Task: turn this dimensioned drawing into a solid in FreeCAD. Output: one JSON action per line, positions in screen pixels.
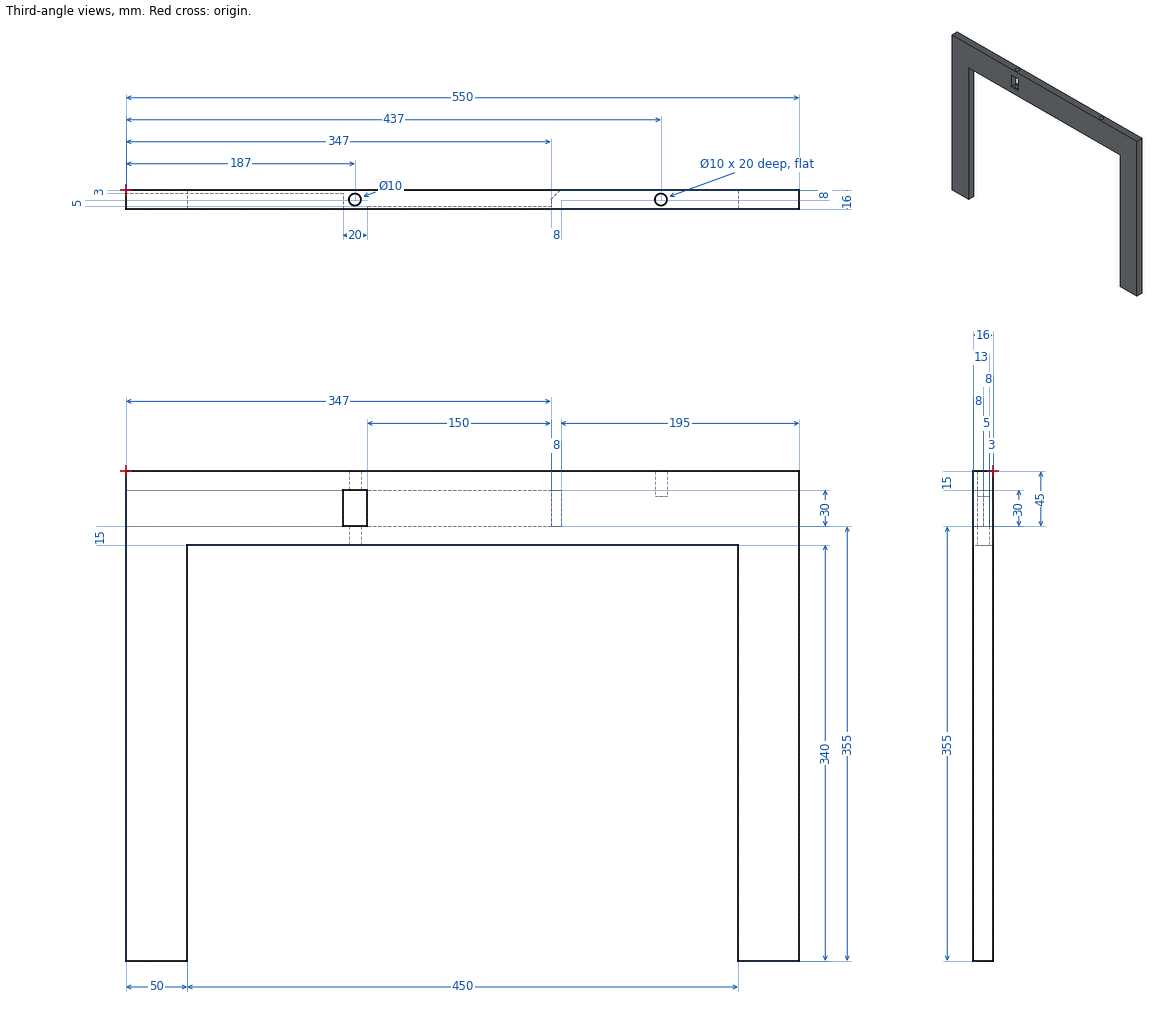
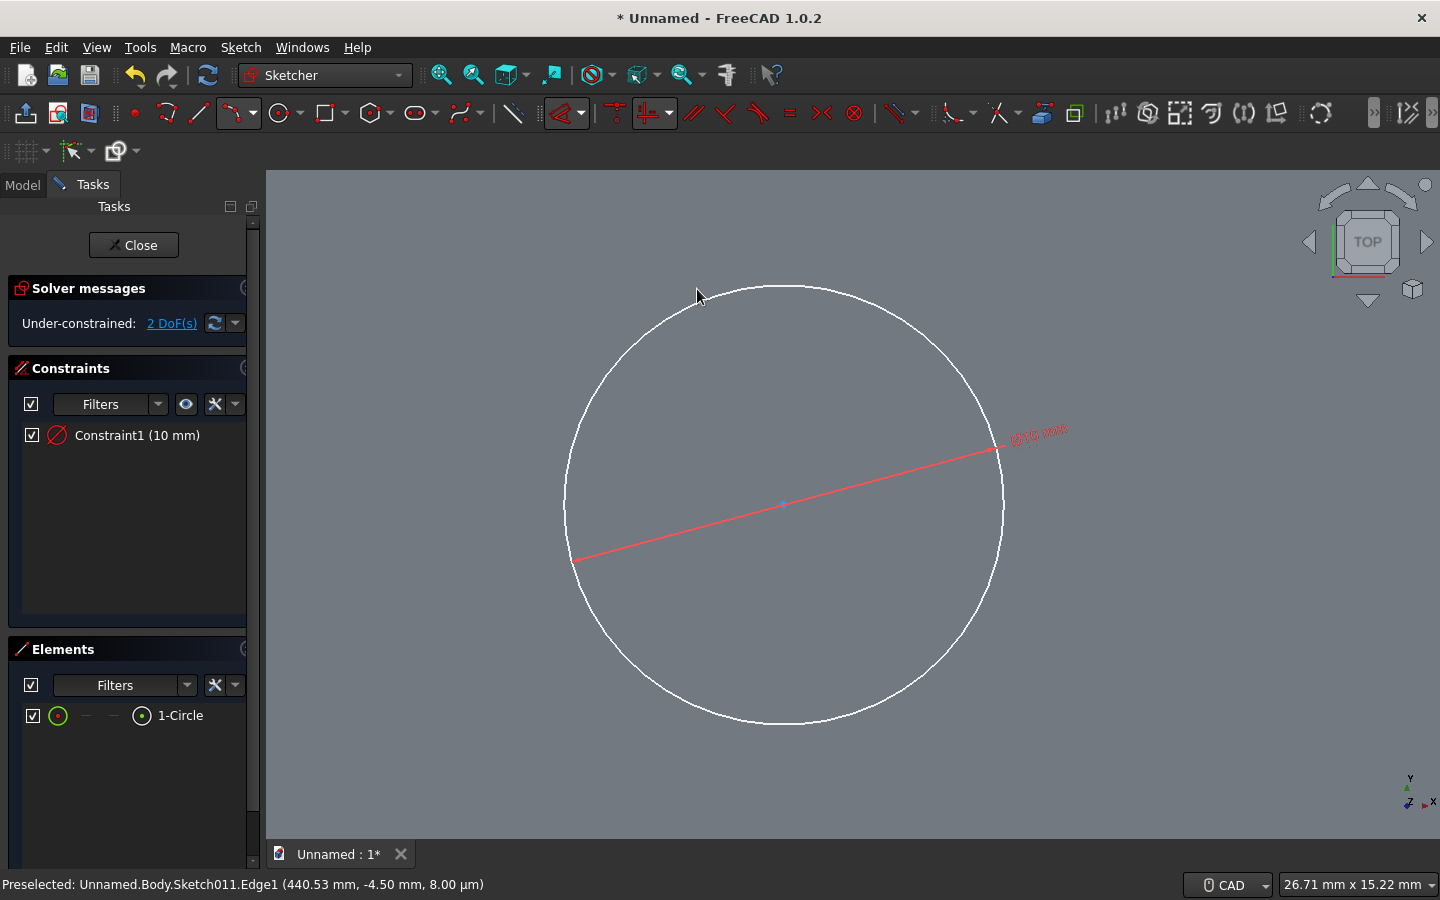
{"action": "left_click", "coordinate": [784, 505]}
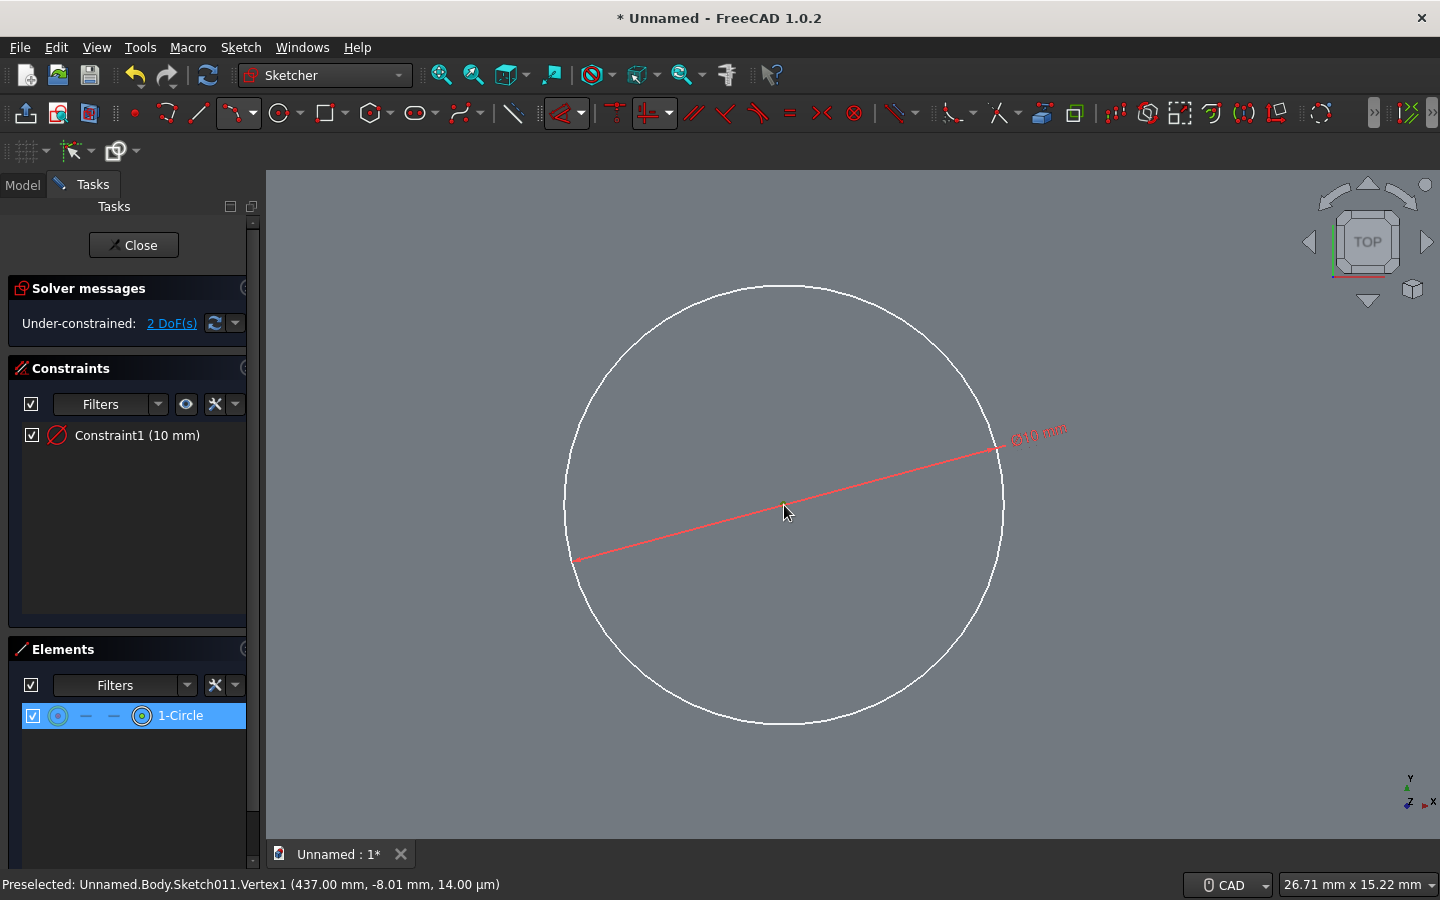
{"action": "left_click", "coordinate": [584, 114]}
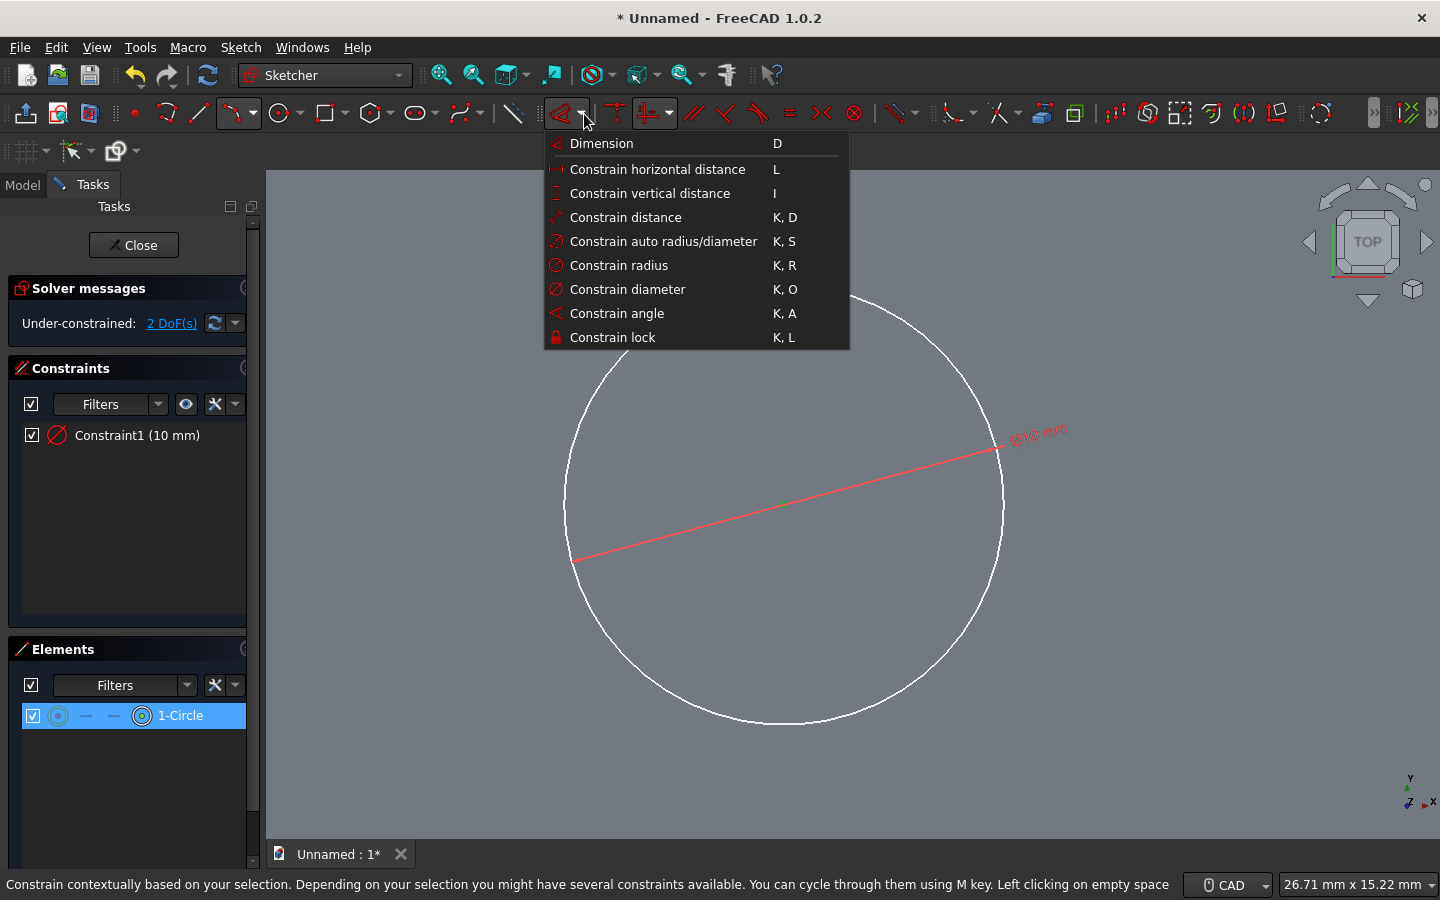
{"action": "left_click", "coordinate": [697, 193]}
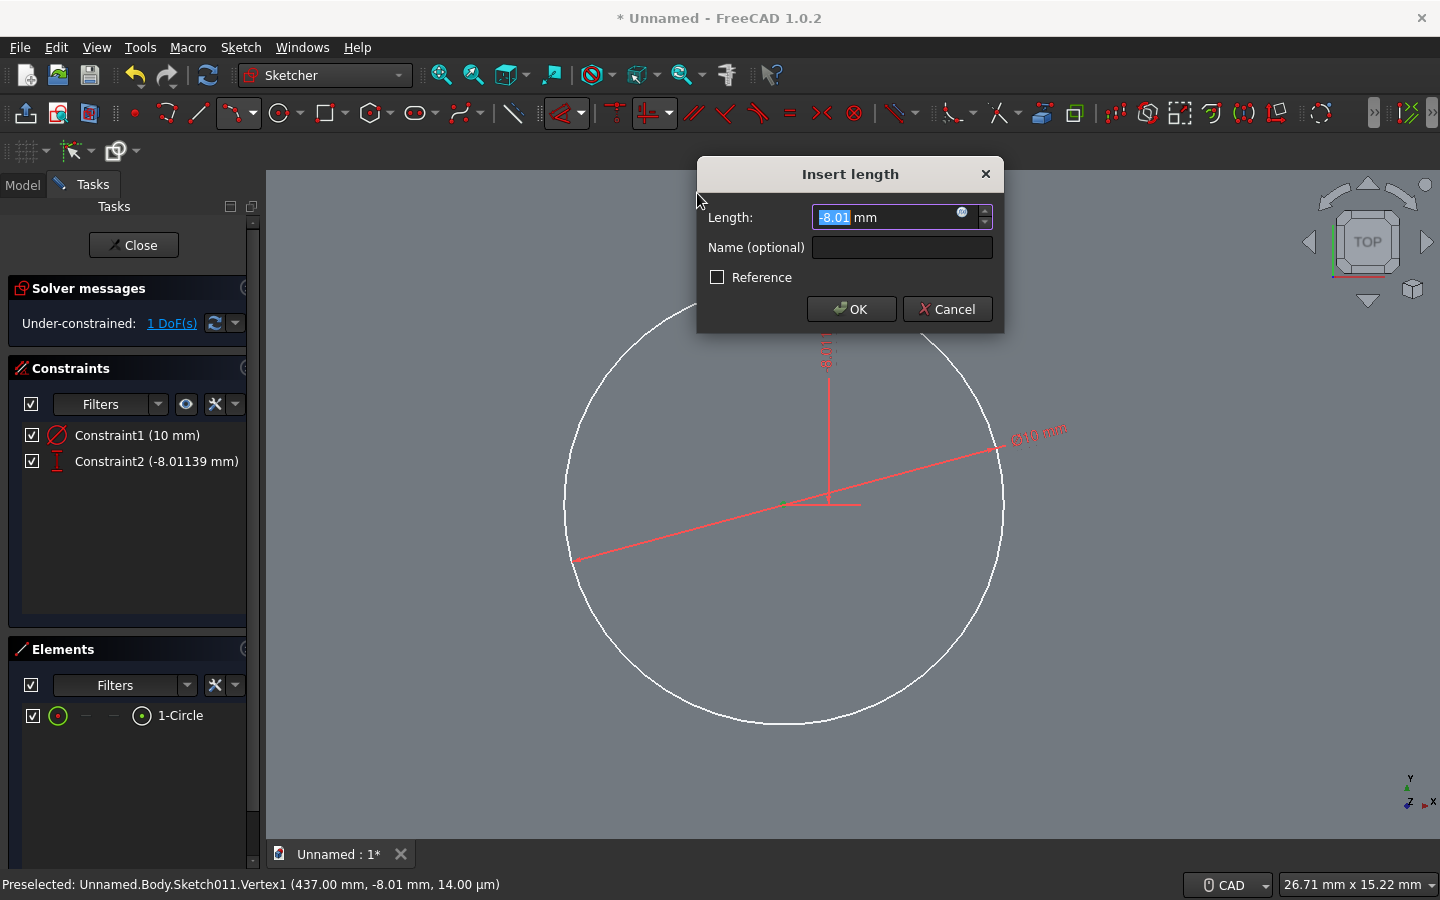
{"action": "type", "text": "-8"}
{"action": "key", "text": "Return"}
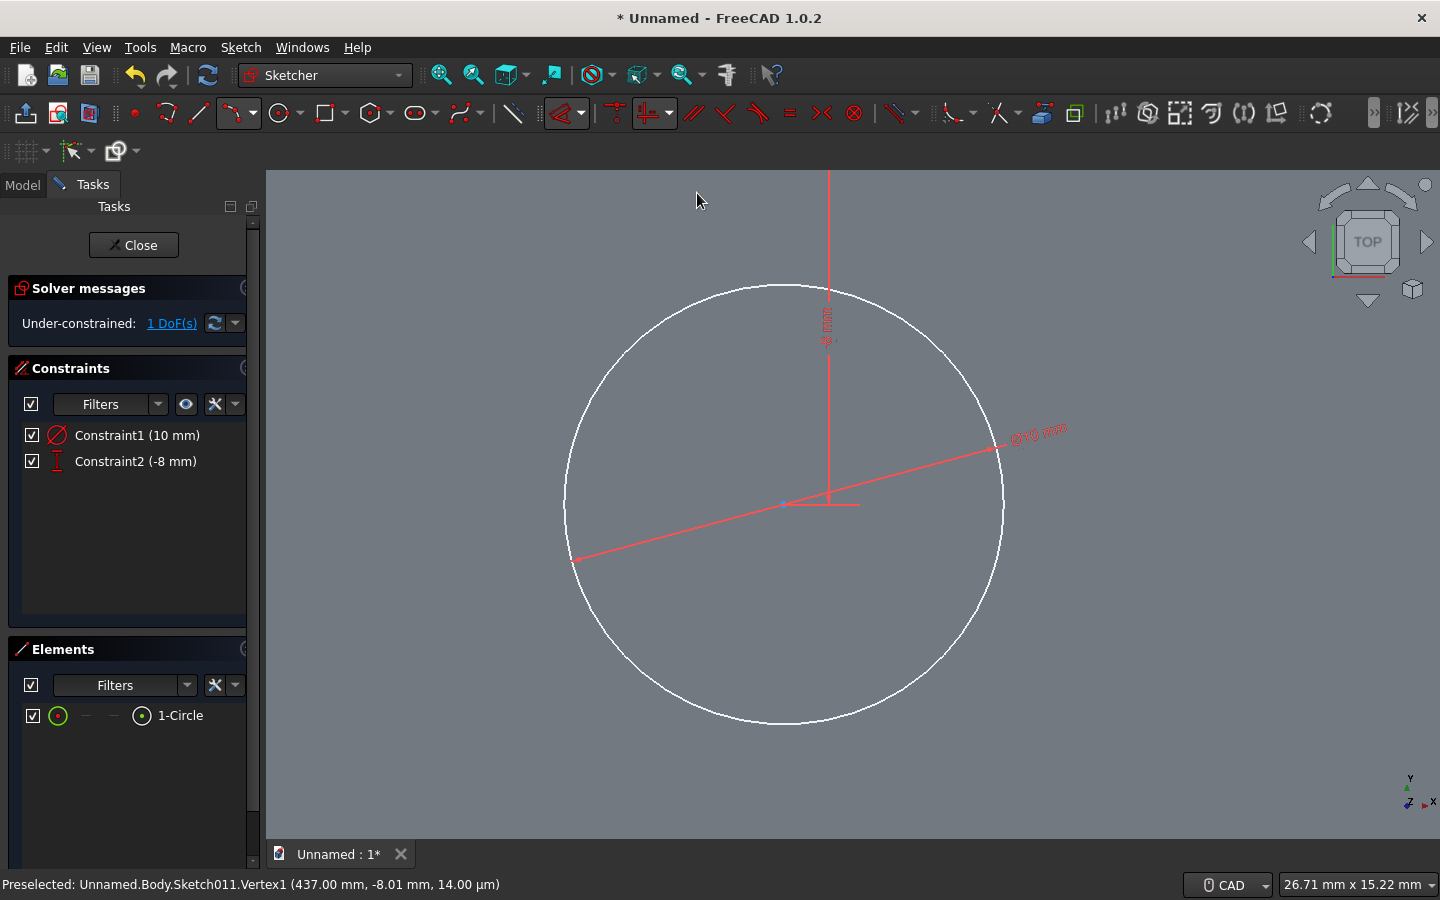
{"action": "left_click", "coordinate": [784, 504]}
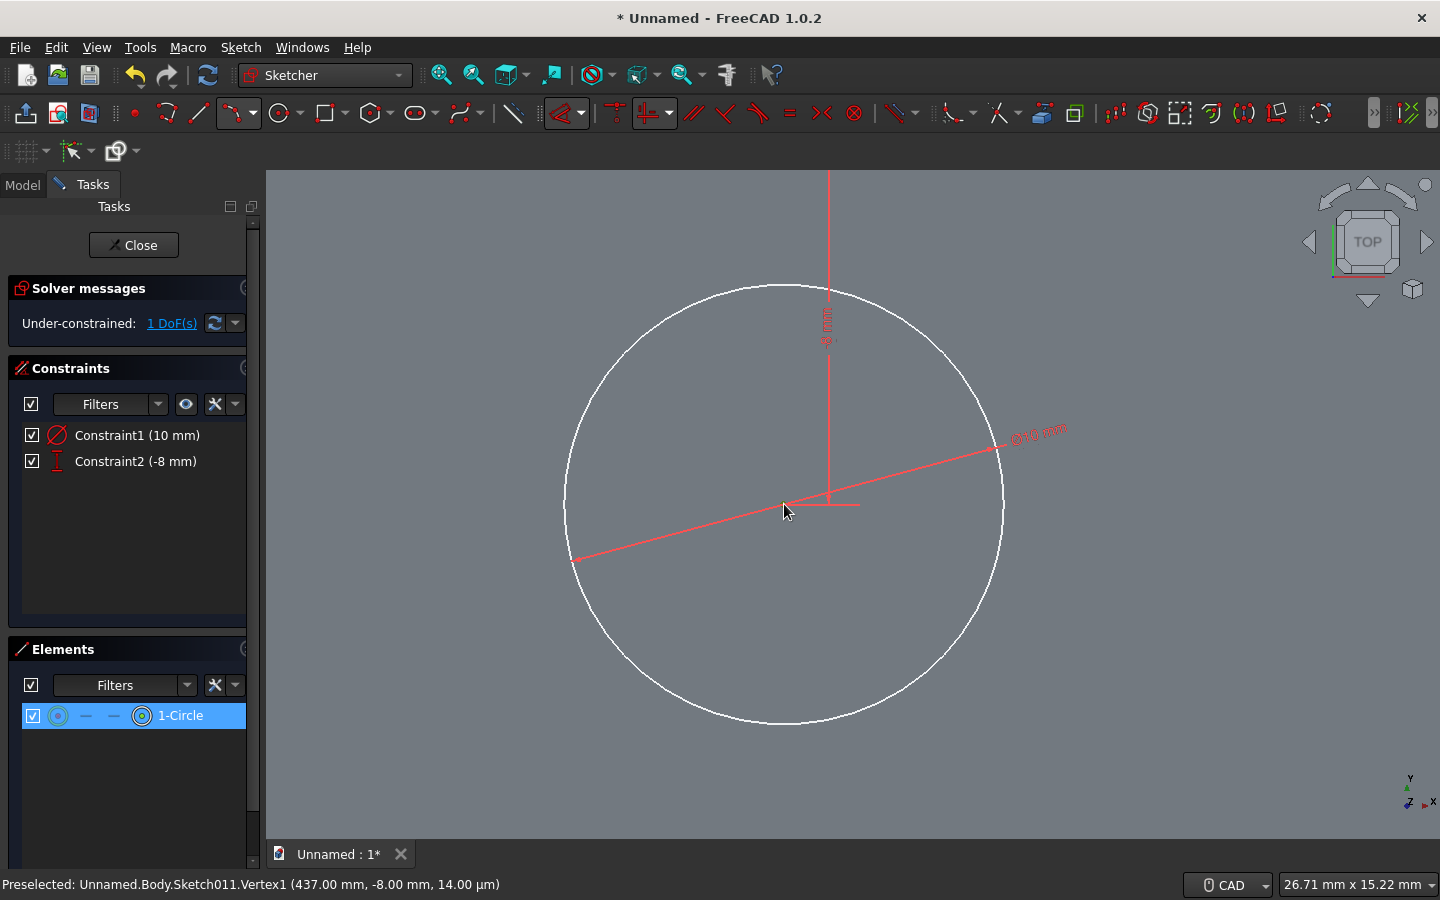
{"action": "left_click", "coordinate": [584, 114]}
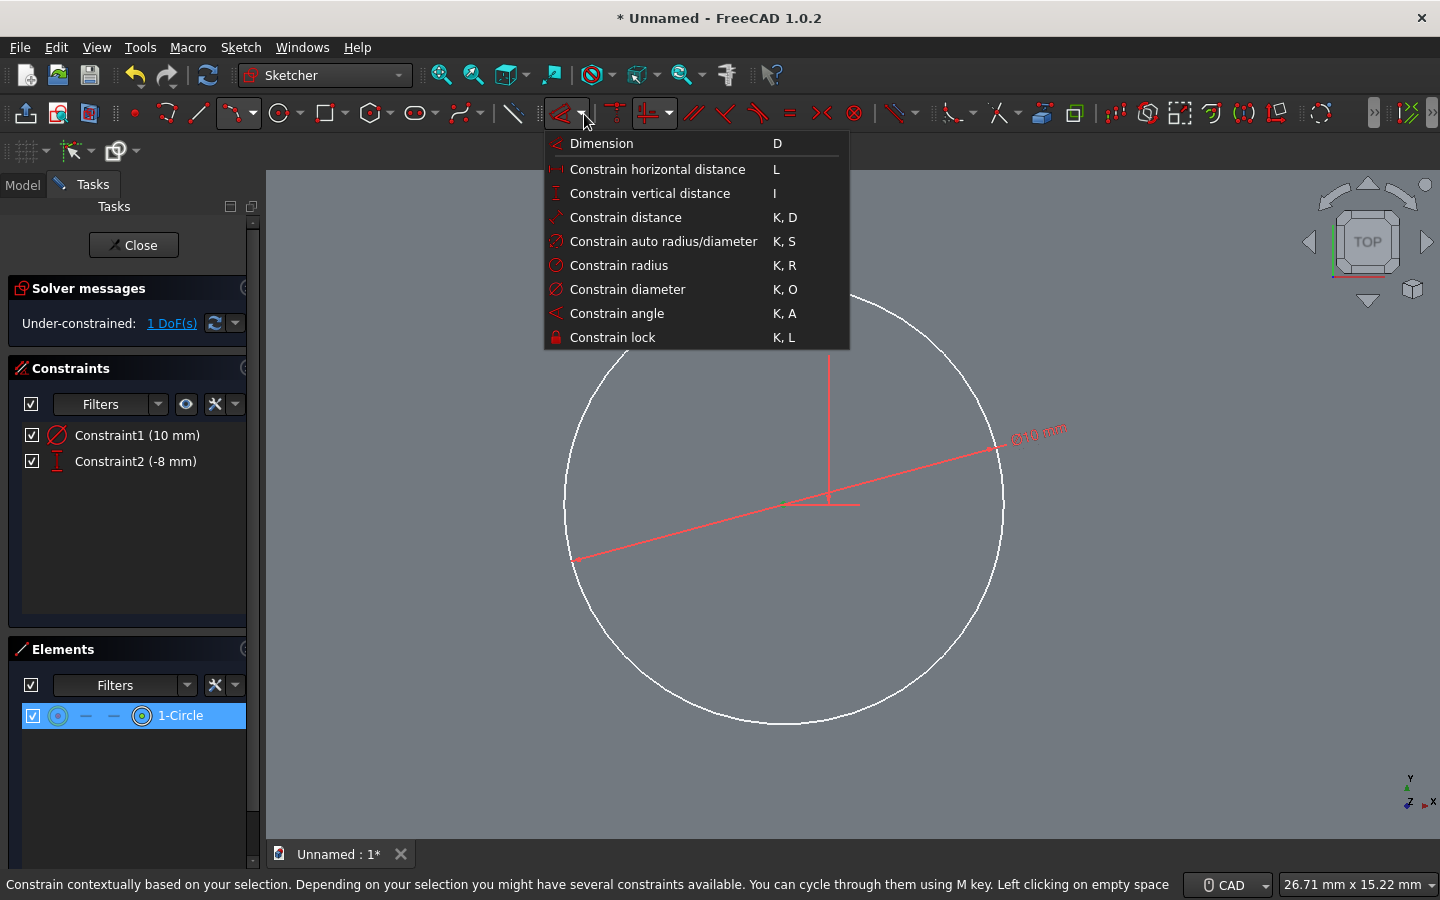
{"action": "left_click", "coordinate": [697, 169]}